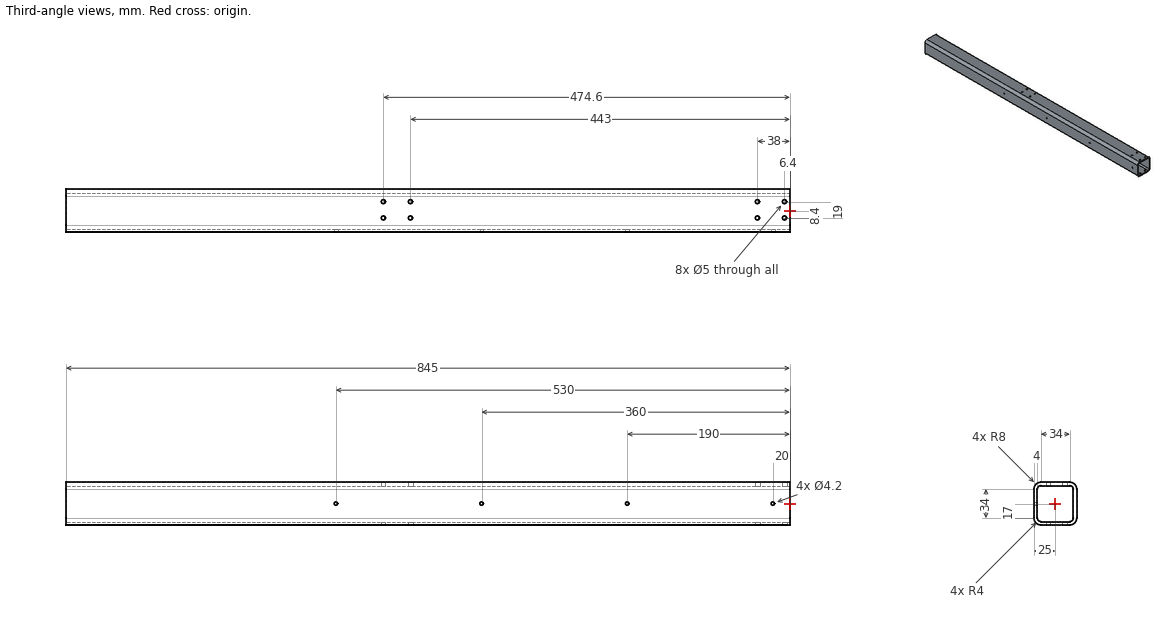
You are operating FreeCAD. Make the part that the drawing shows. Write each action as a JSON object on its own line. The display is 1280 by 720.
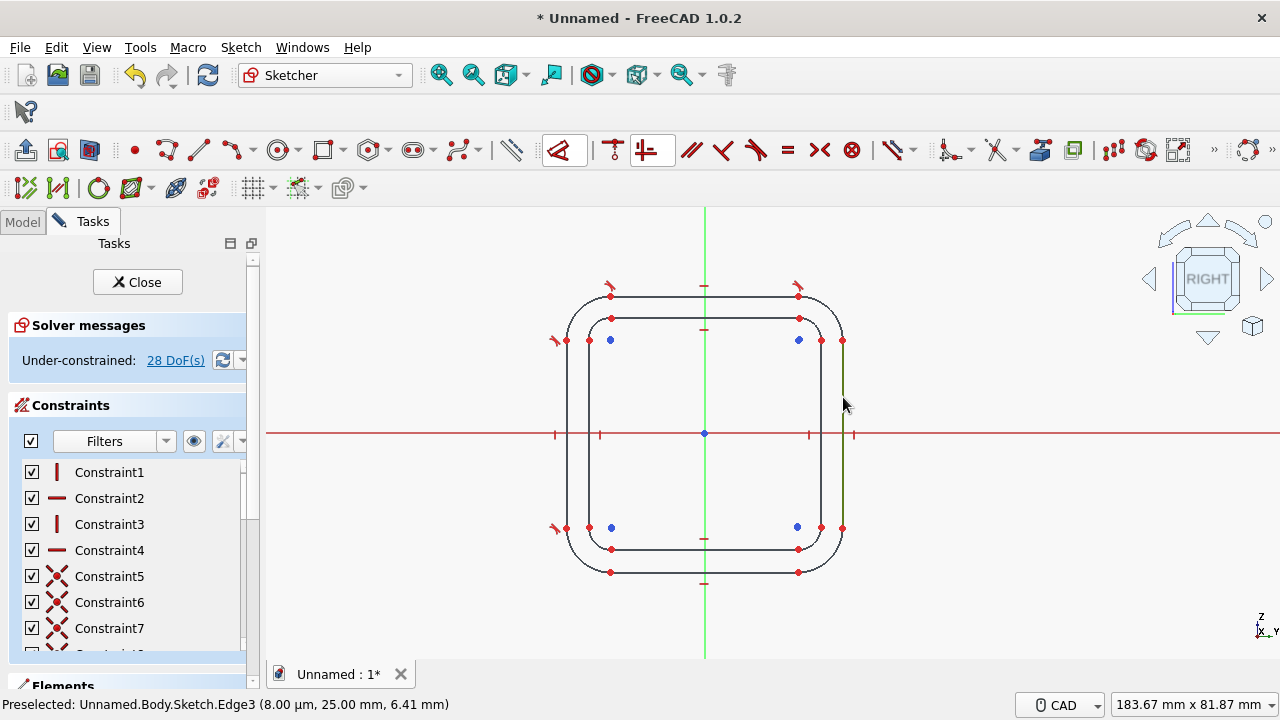
{"action": "left_click", "coordinate": [838, 321]}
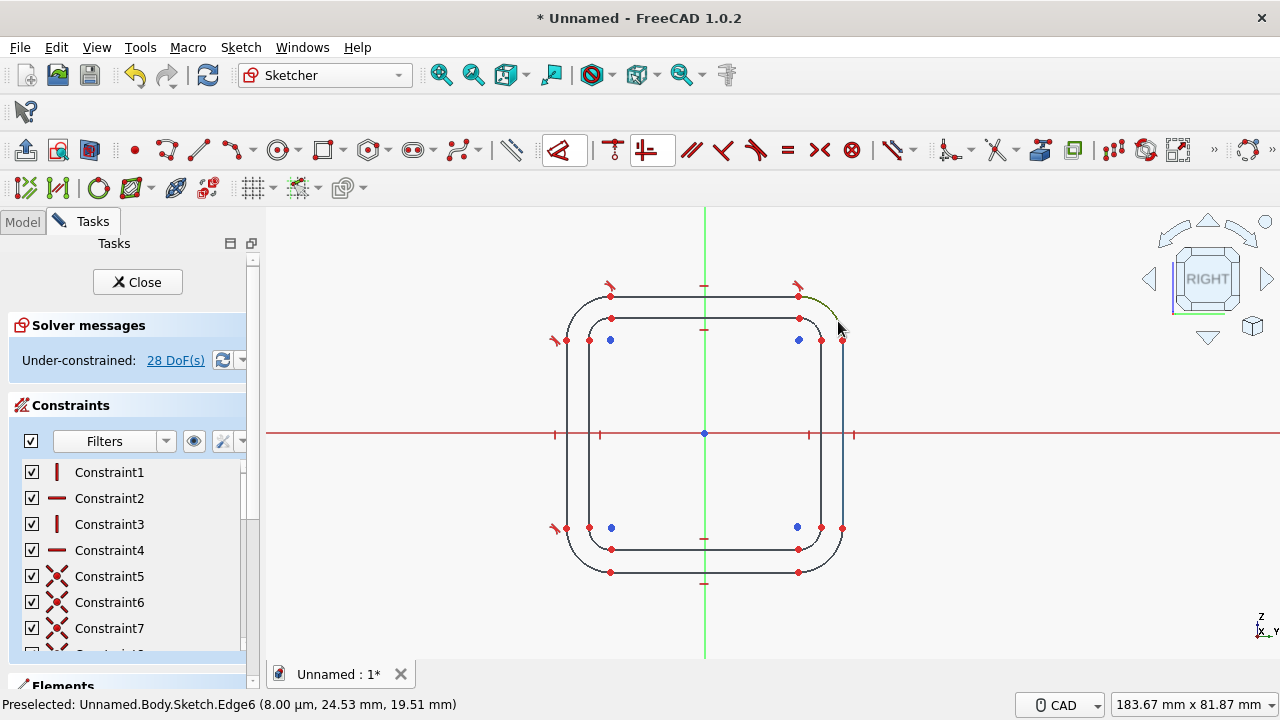
{"action": "left_click", "coordinate": [756, 150]}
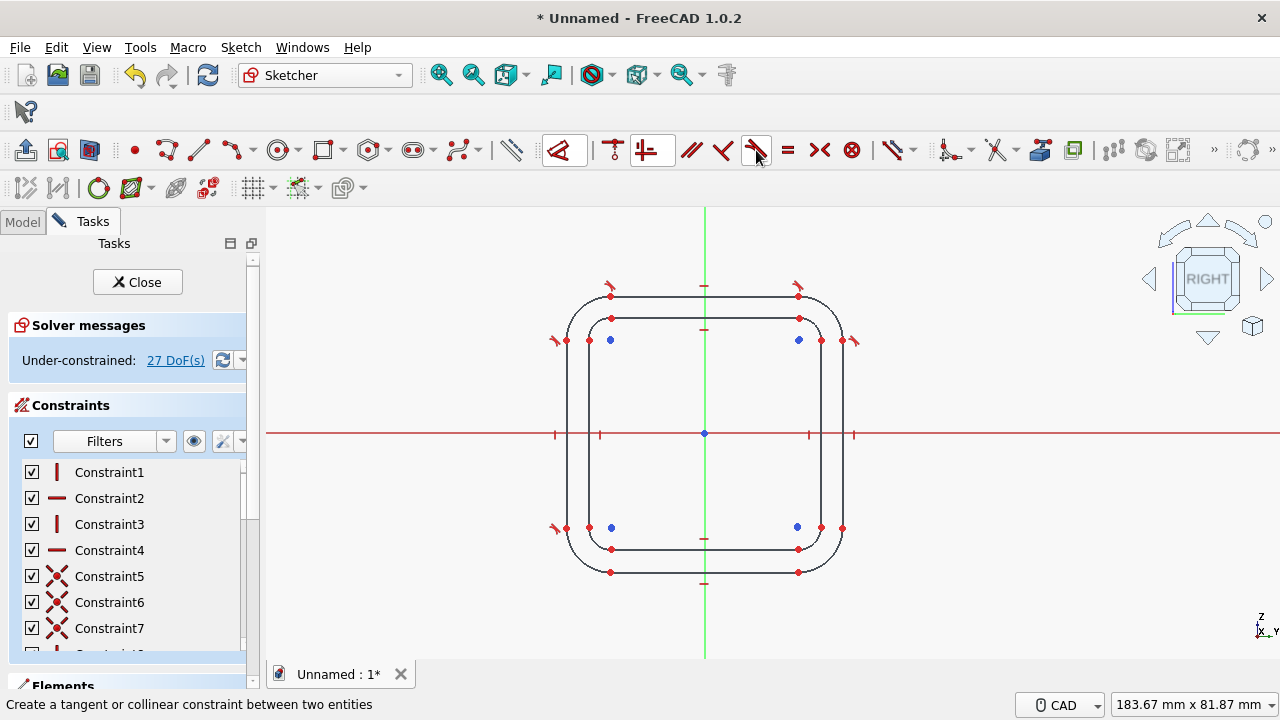
{"action": "left_click", "coordinate": [843, 397]}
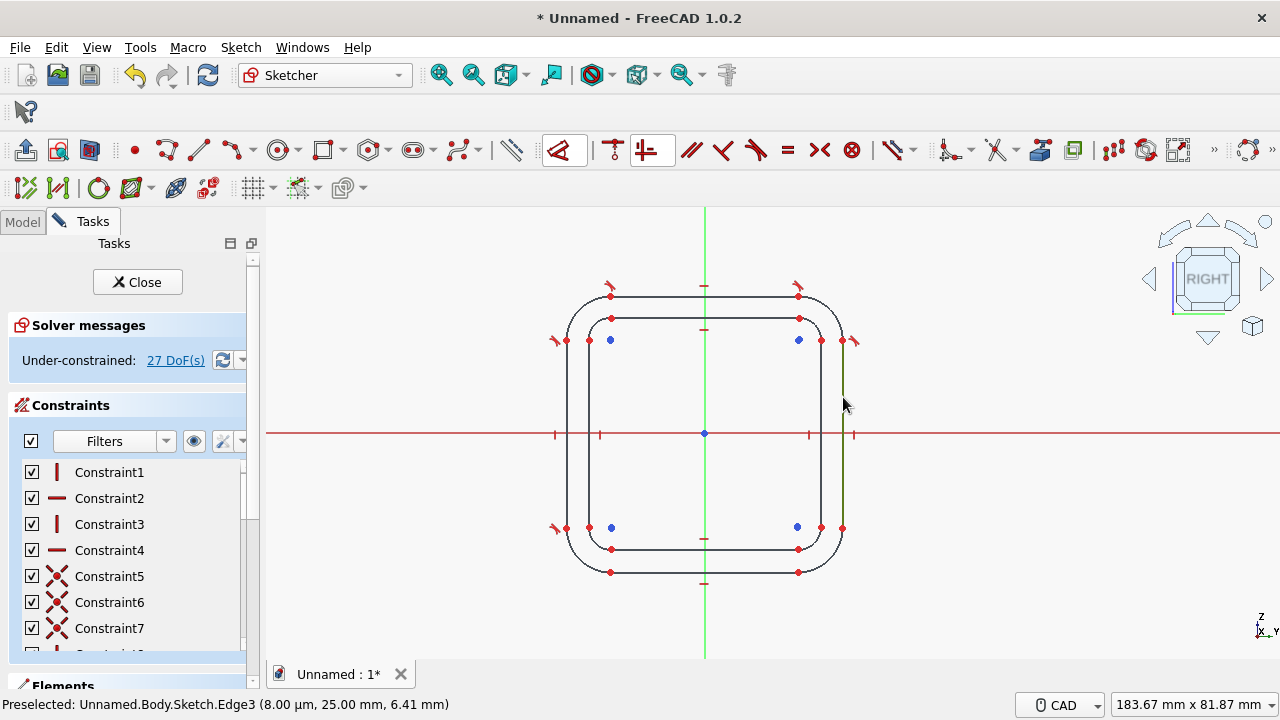
{"action": "left_click", "coordinate": [818, 567]}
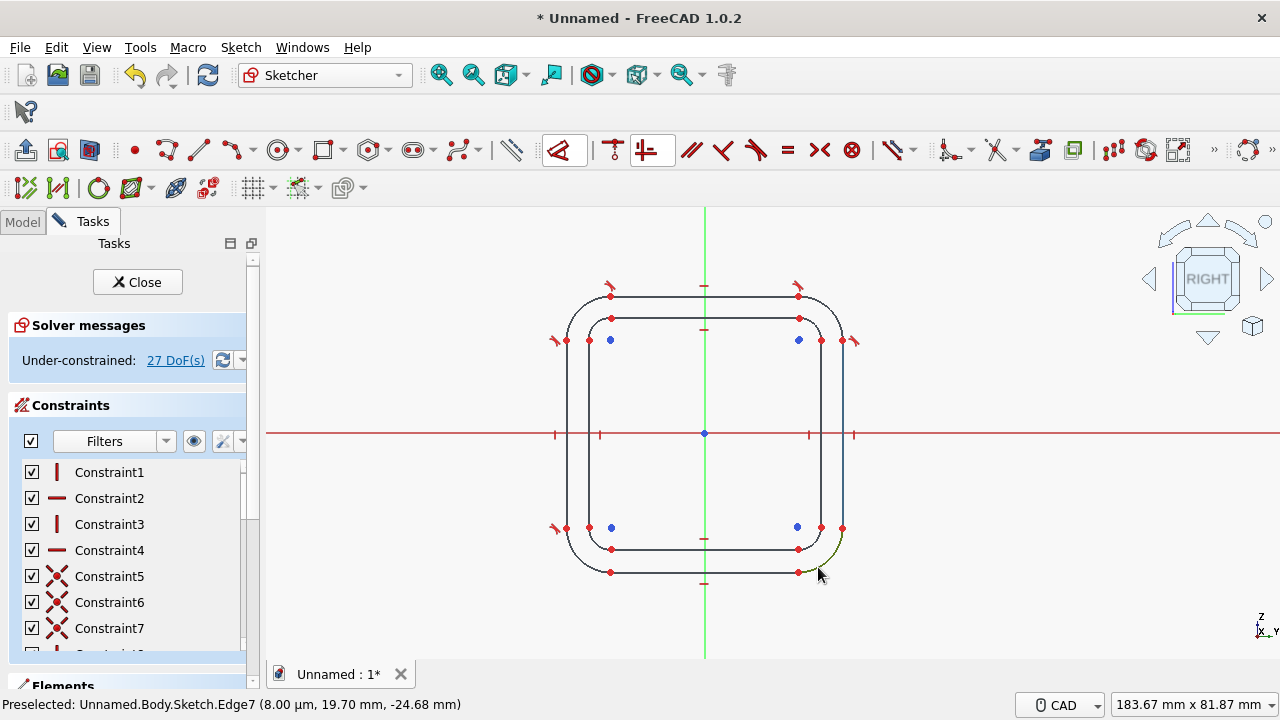
{"action": "left_click", "coordinate": [756, 150]}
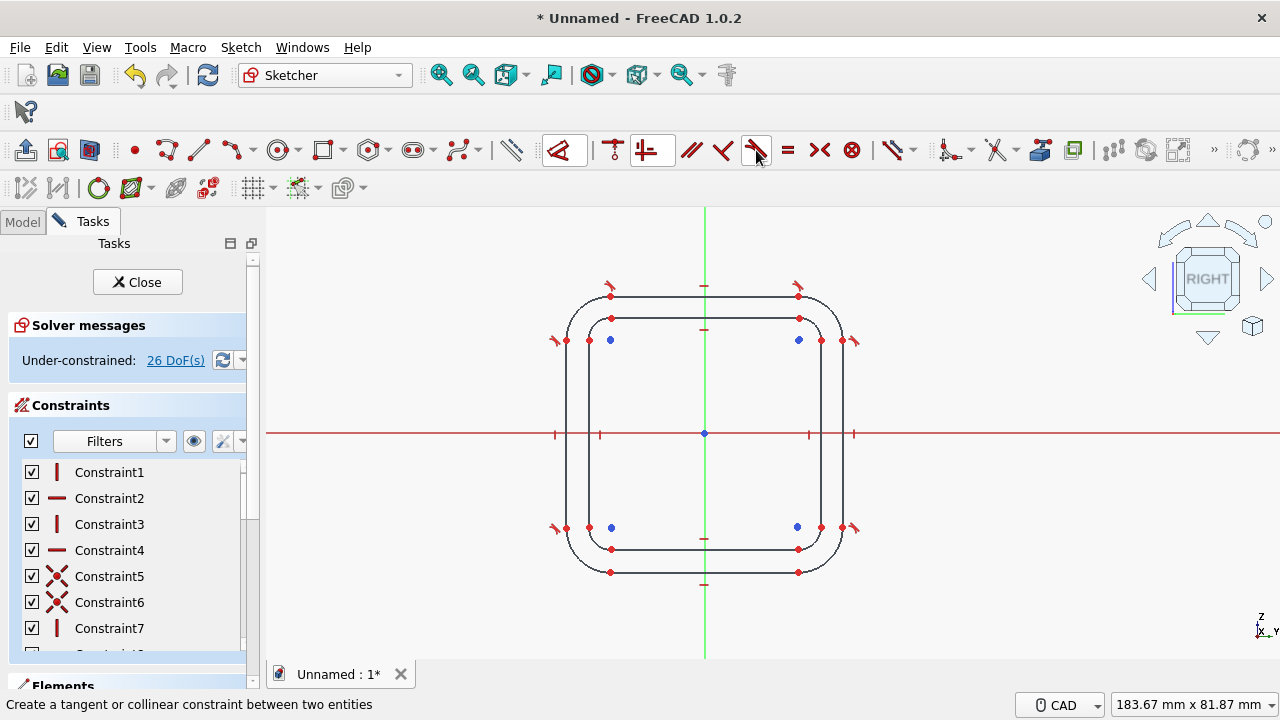
{"action": "left_click", "coordinate": [742, 573]}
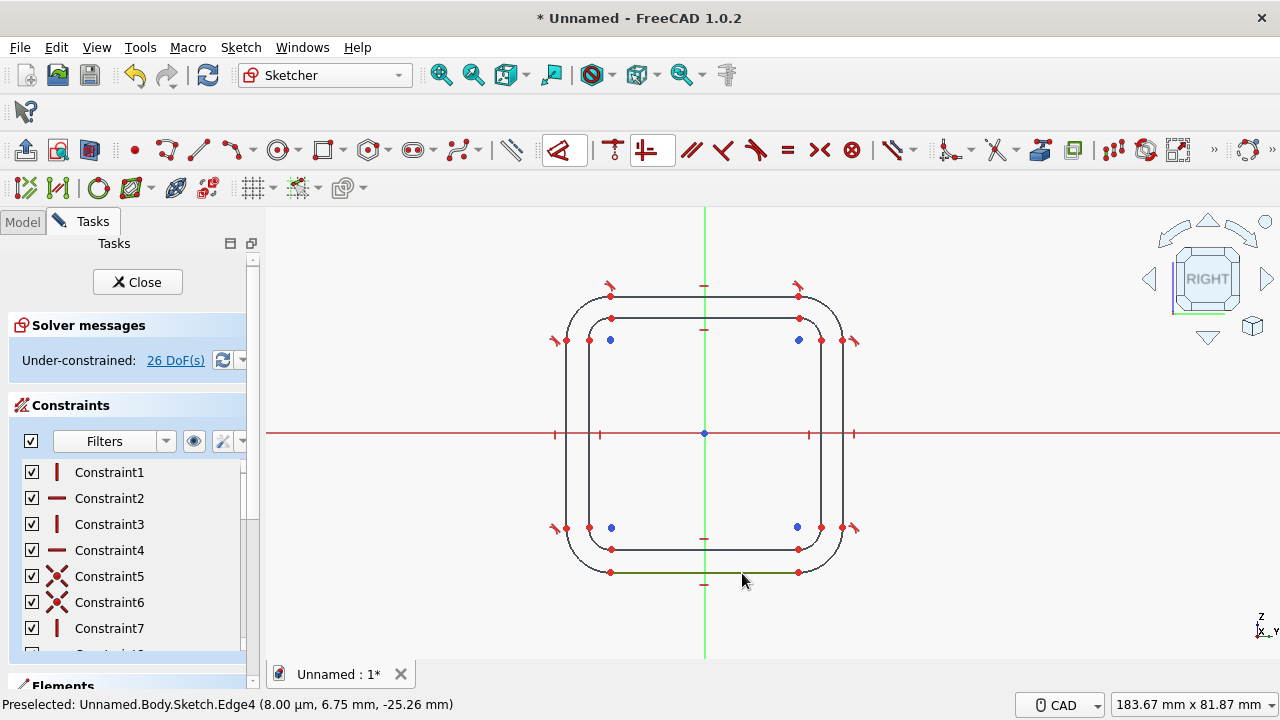
{"action": "left_click", "coordinate": [819, 567]}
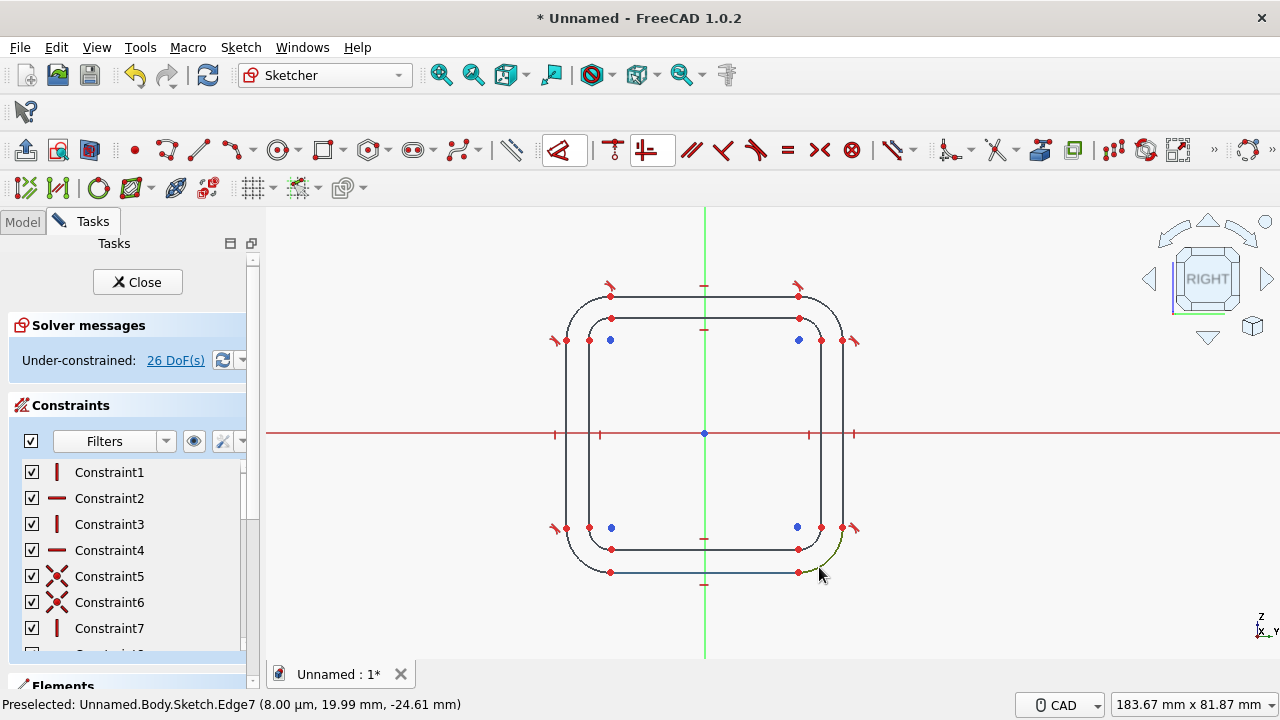
{"action": "left_click", "coordinate": [756, 150]}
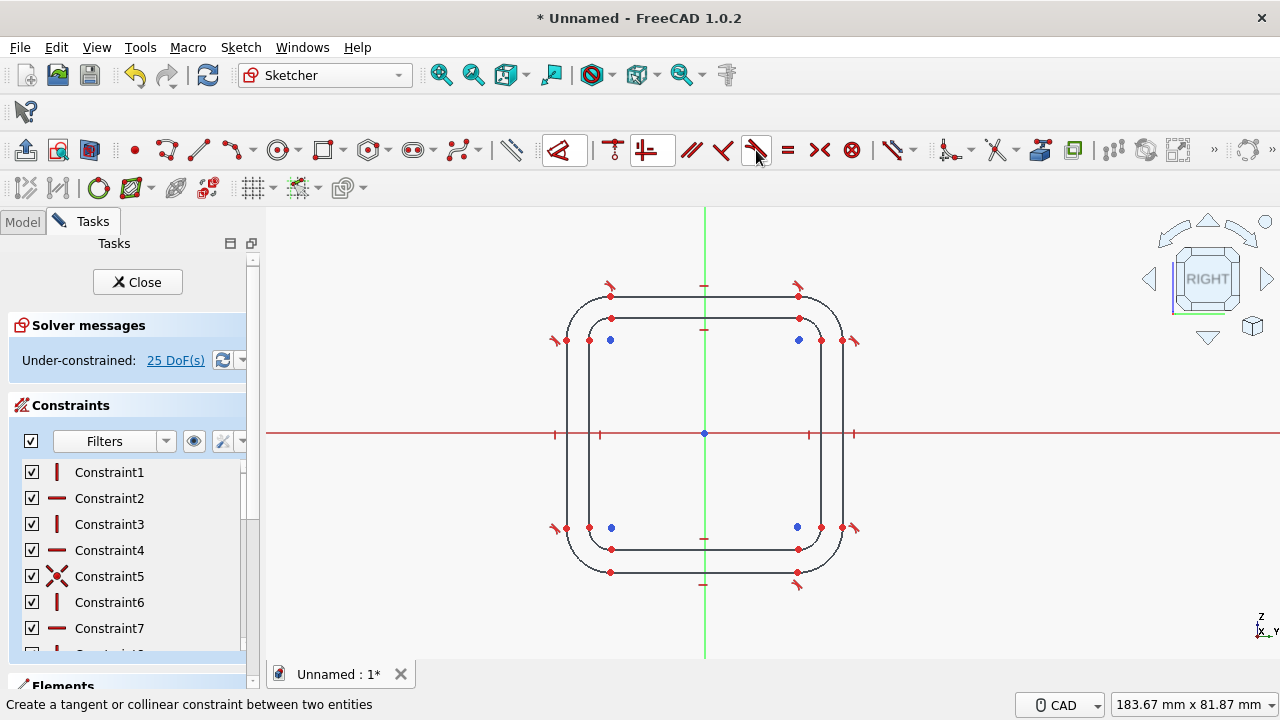
{"action": "left_click", "coordinate": [741, 573]}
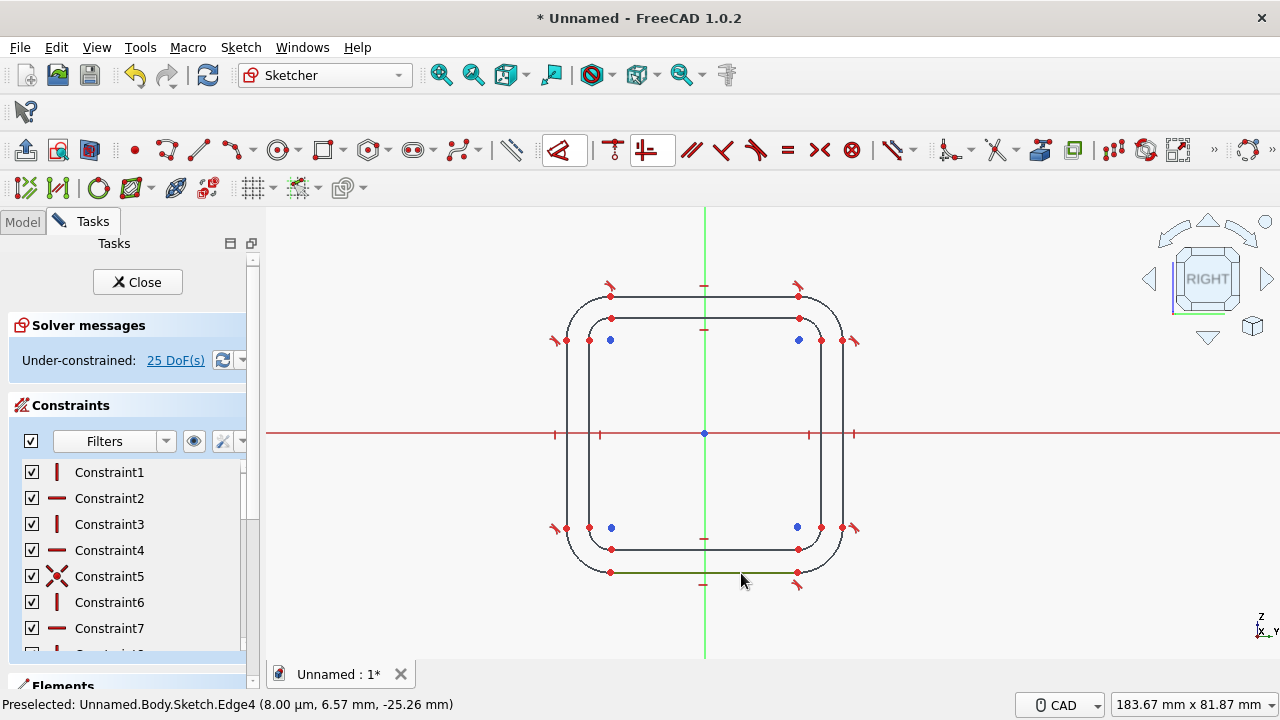
{"action": "left_click", "coordinate": [571, 548]}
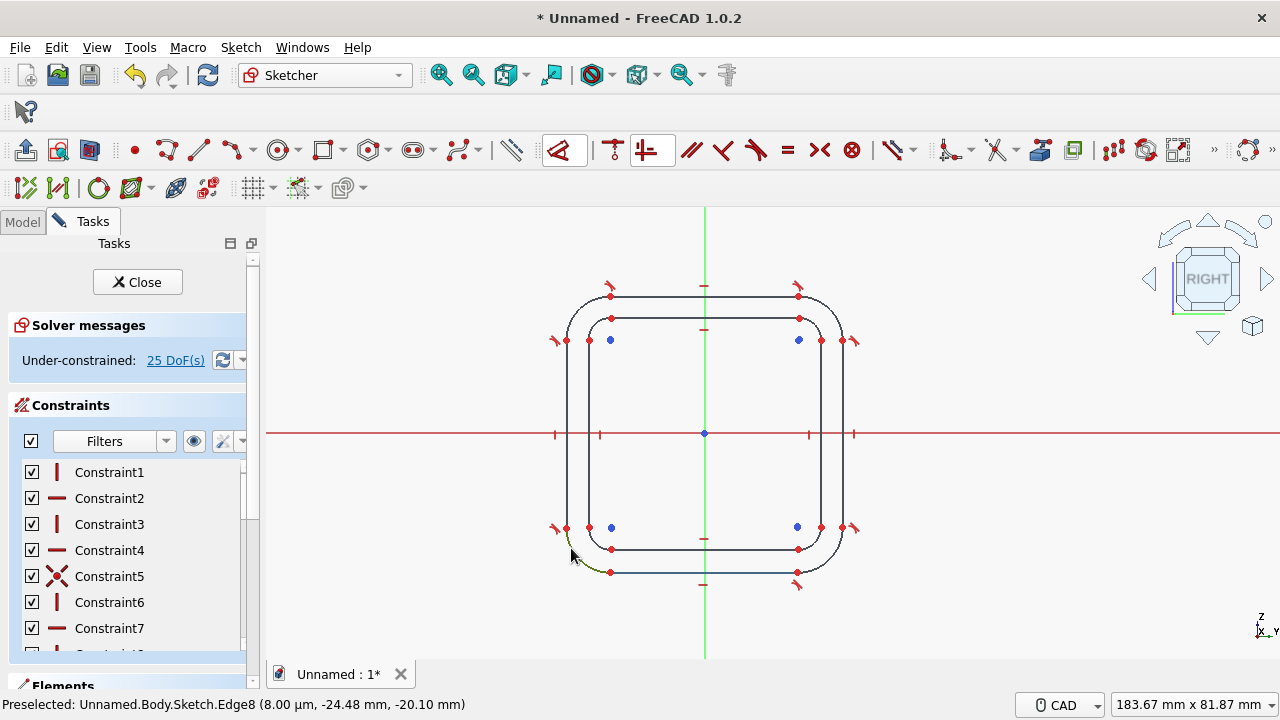
{"action": "left_click", "coordinate": [756, 150]}